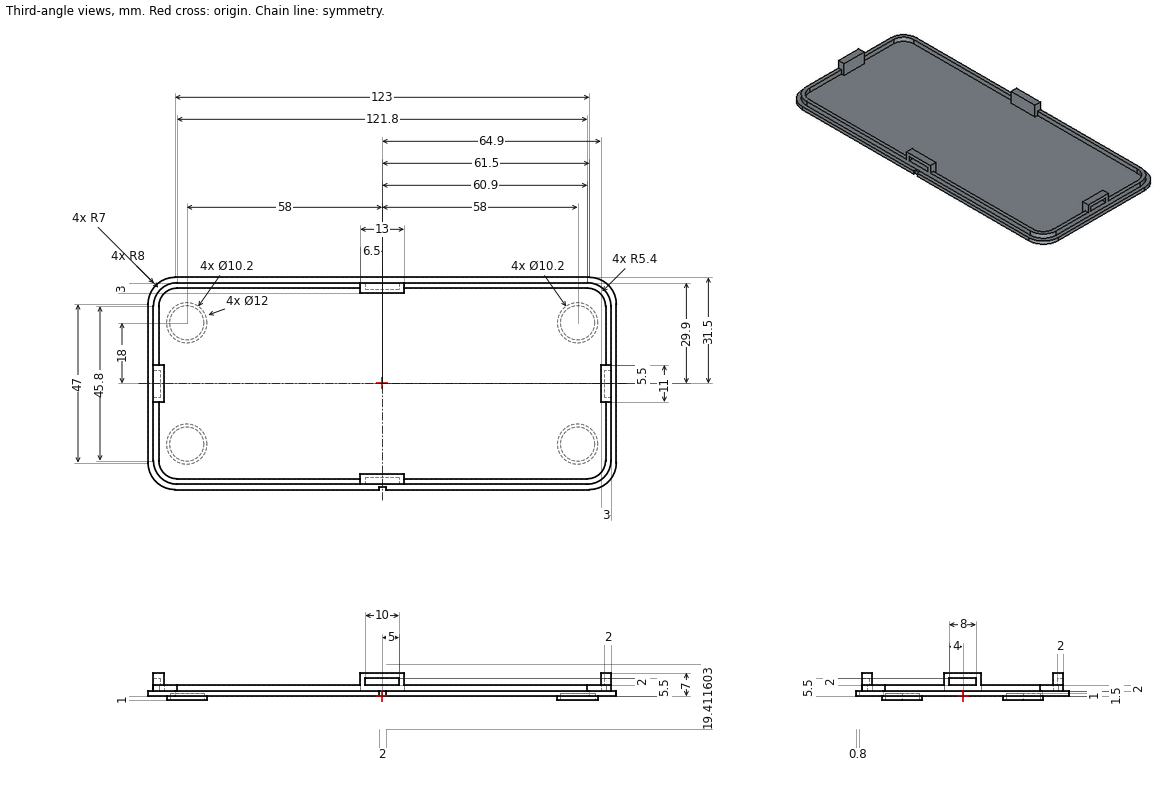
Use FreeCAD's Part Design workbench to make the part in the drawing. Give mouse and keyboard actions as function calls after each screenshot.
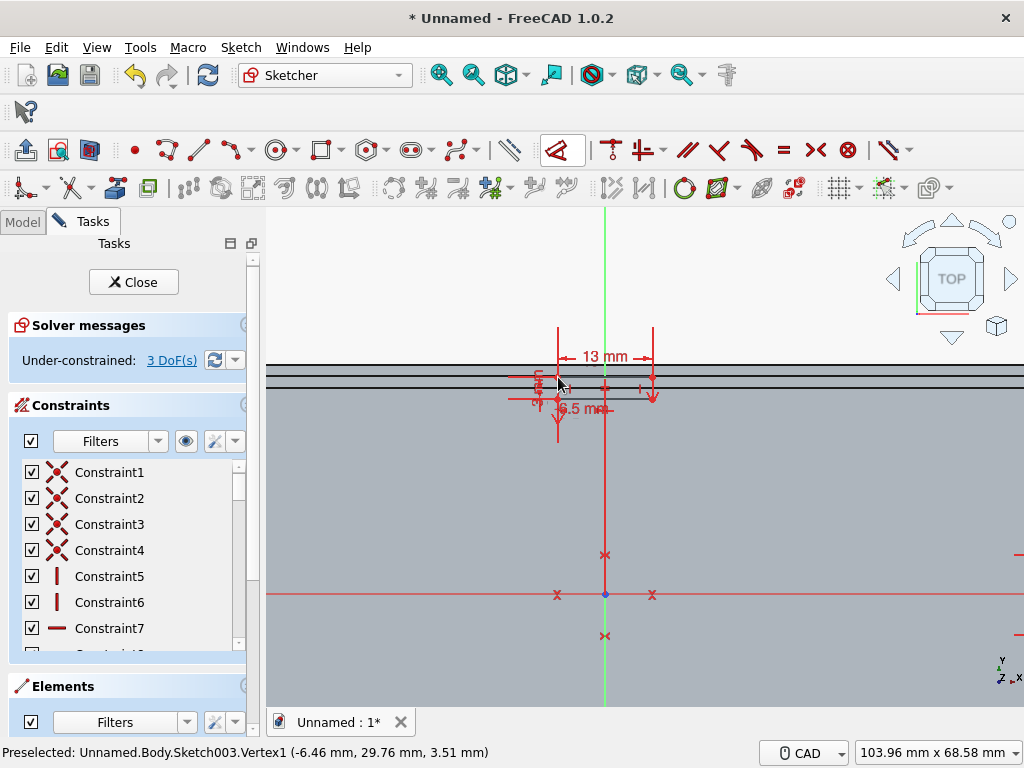
scroll(560, 377, down, 5)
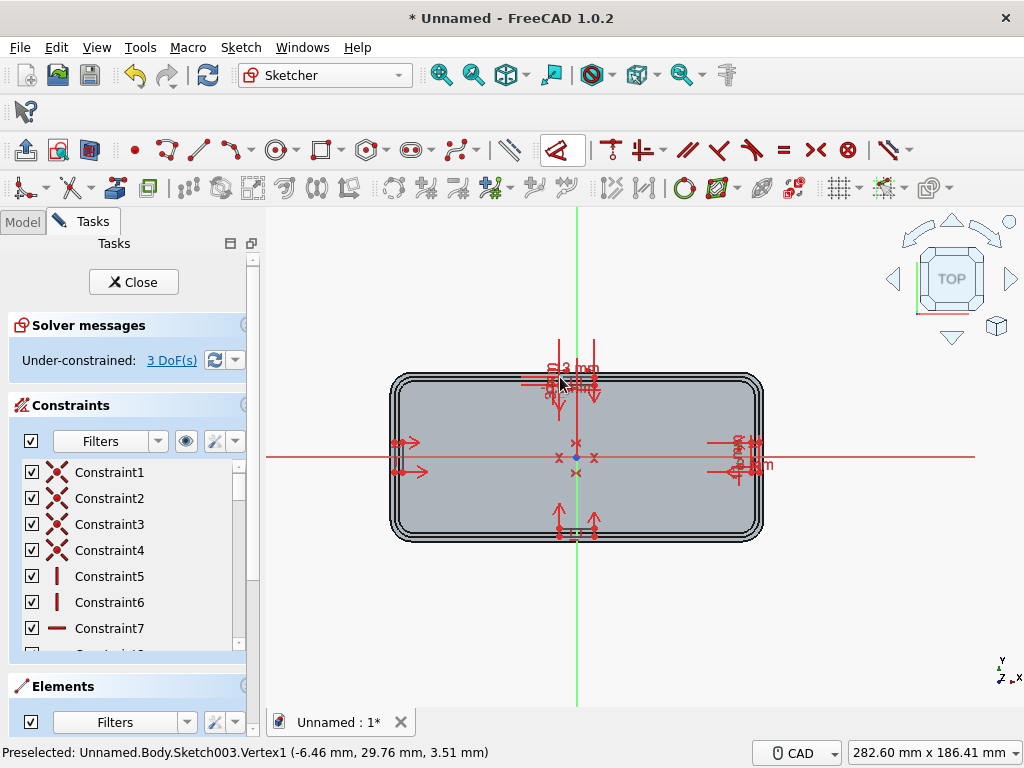
scroll(751, 443, up, 5)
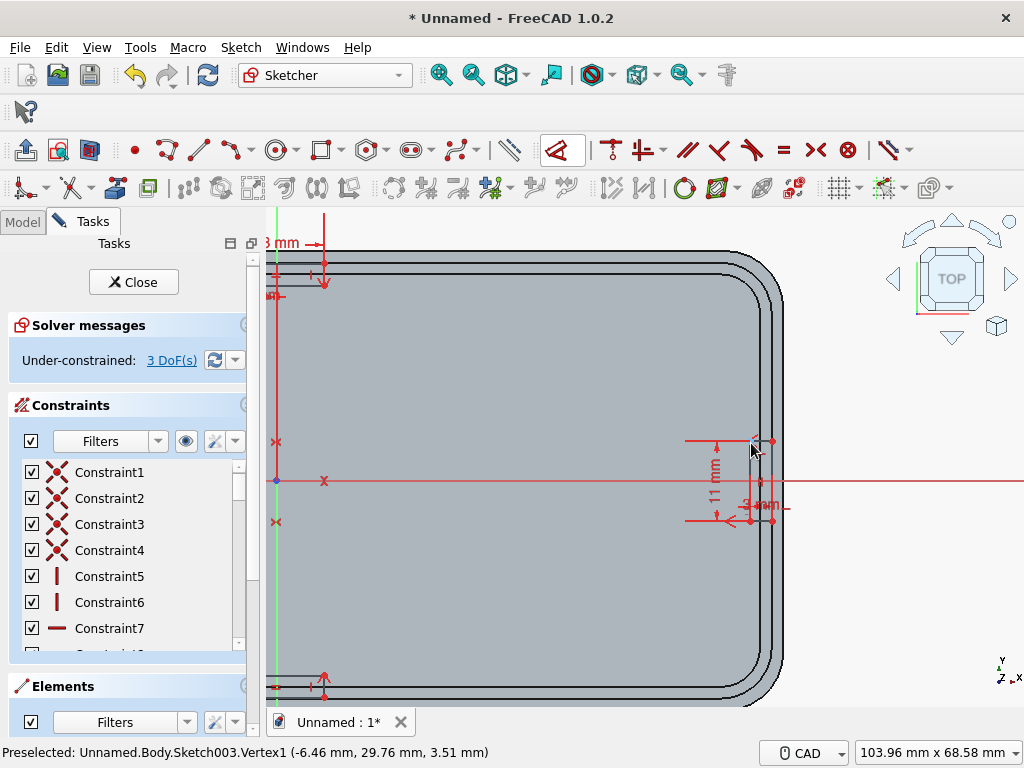
click(750, 441)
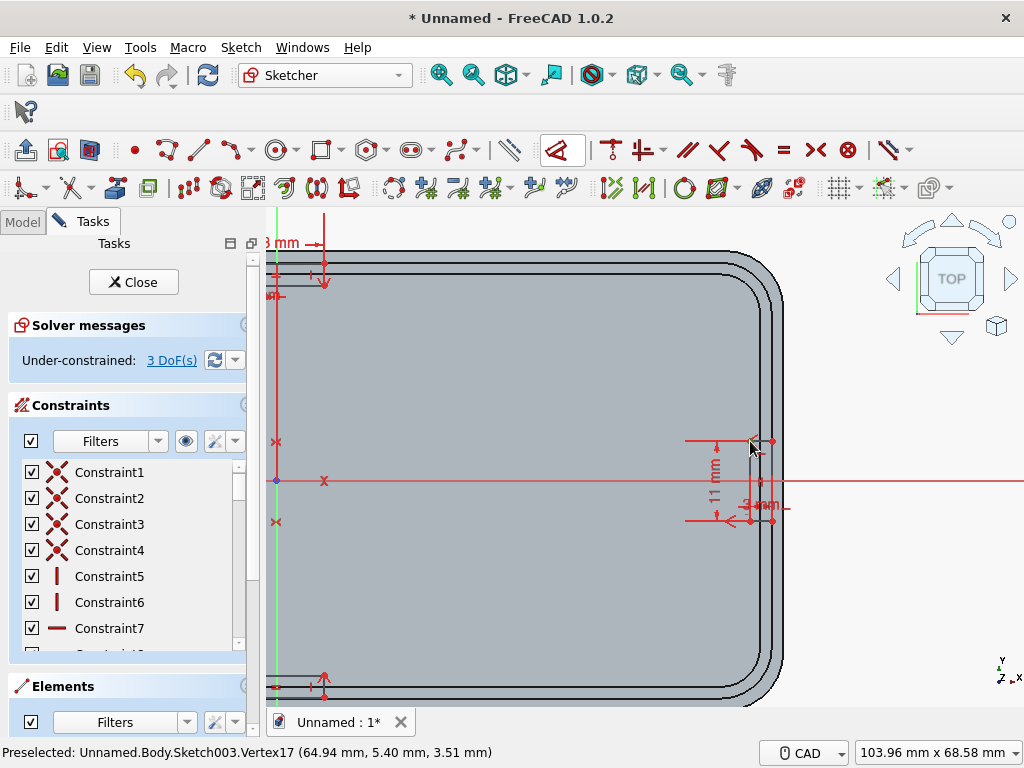
key(i)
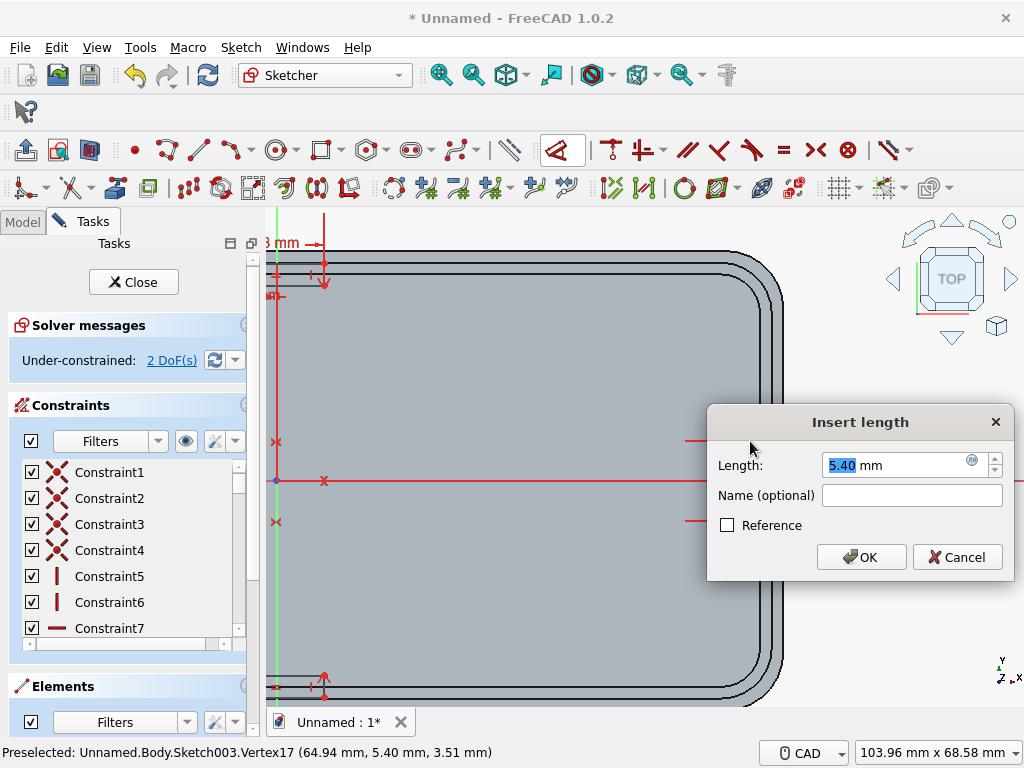
text(5.5)
key(Return)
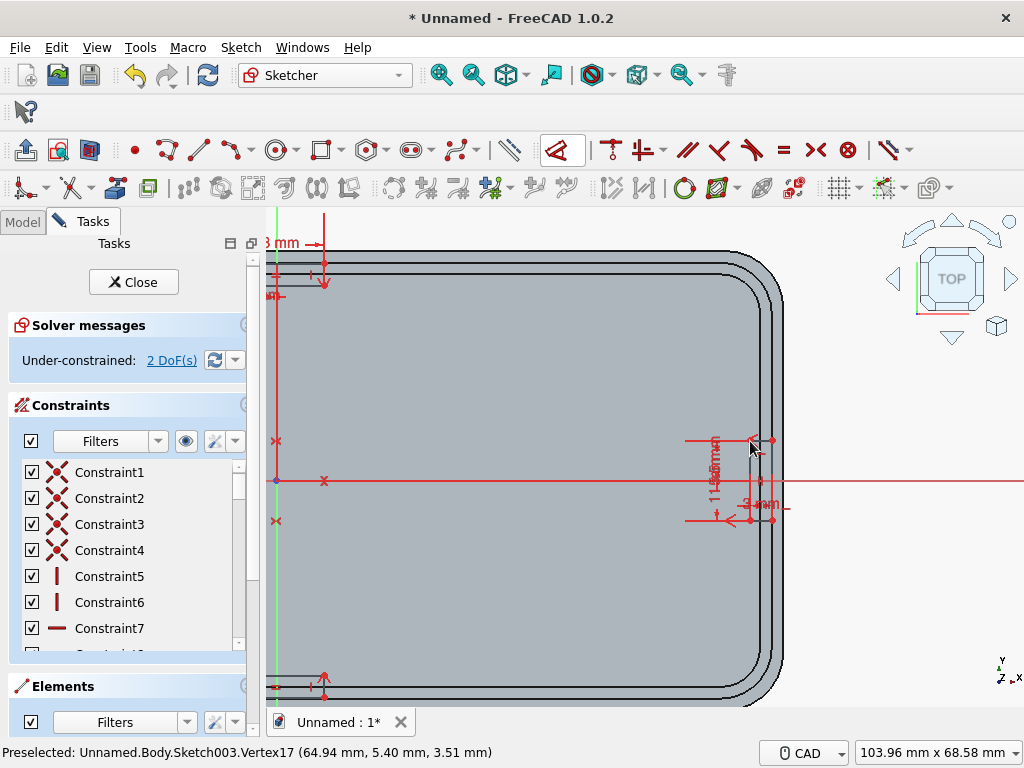
scroll(751, 443, down, 5)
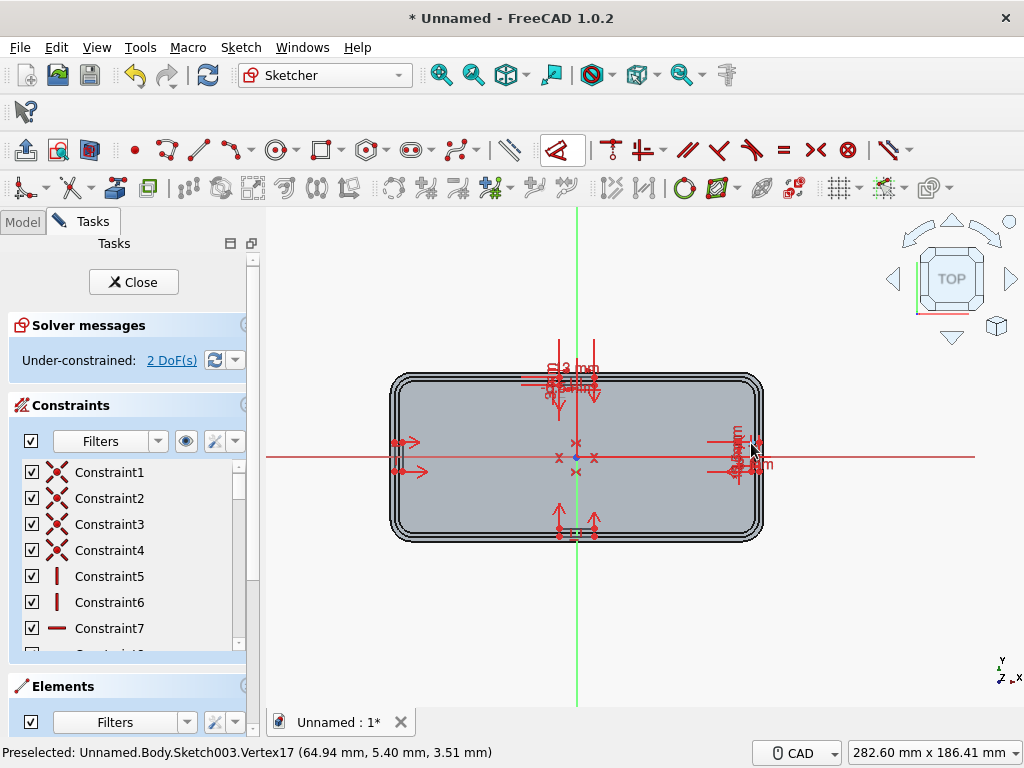
scroll(559, 377, up, 3)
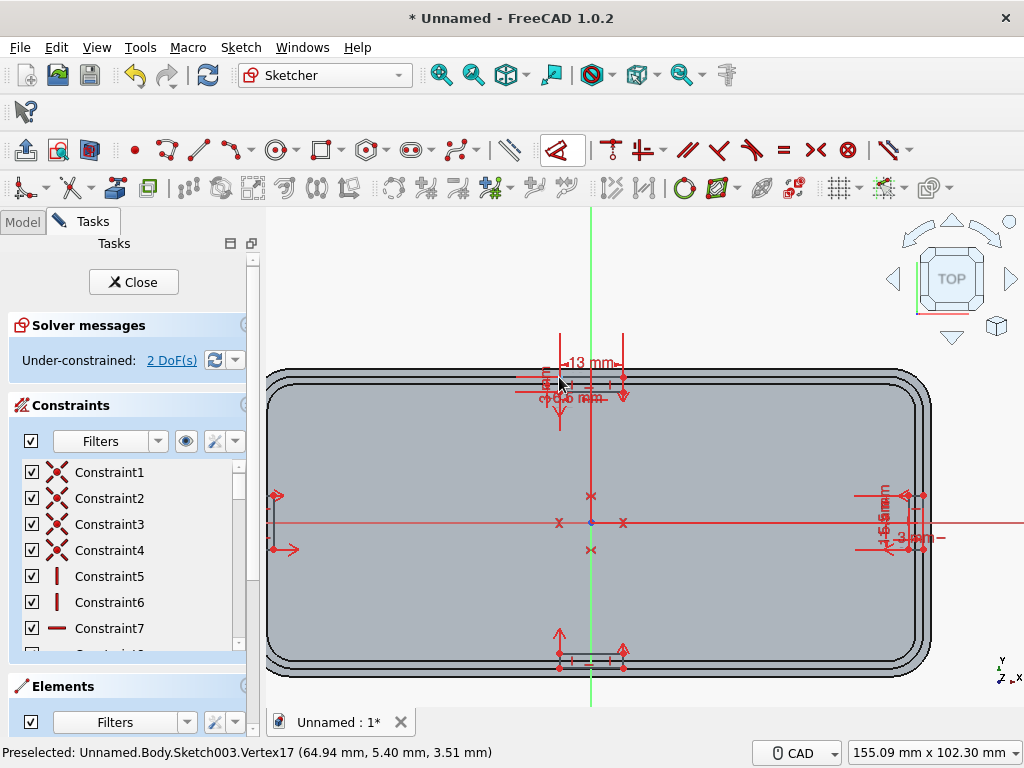
click(560, 377)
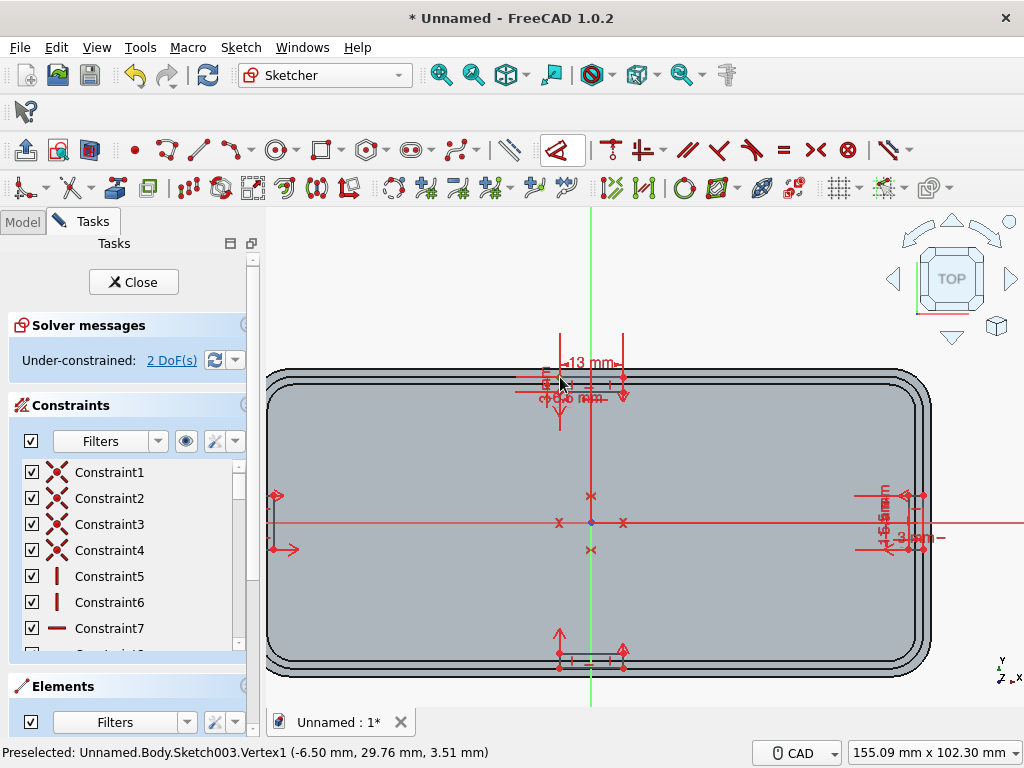
key(i)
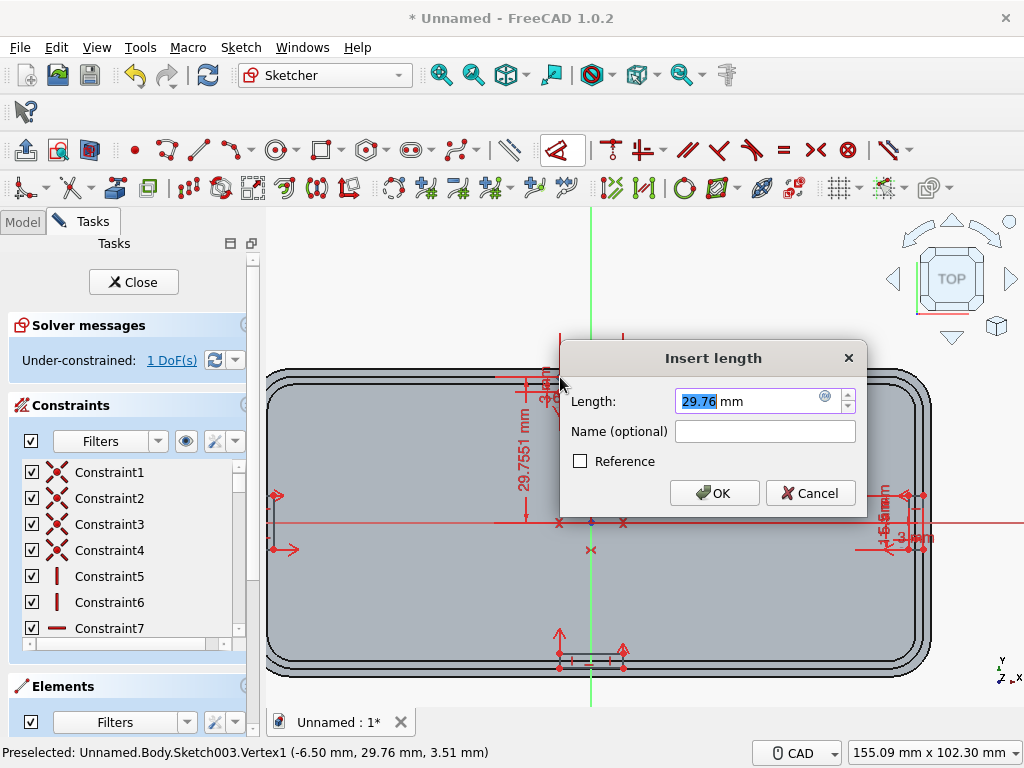
text(29.9)
key(Return)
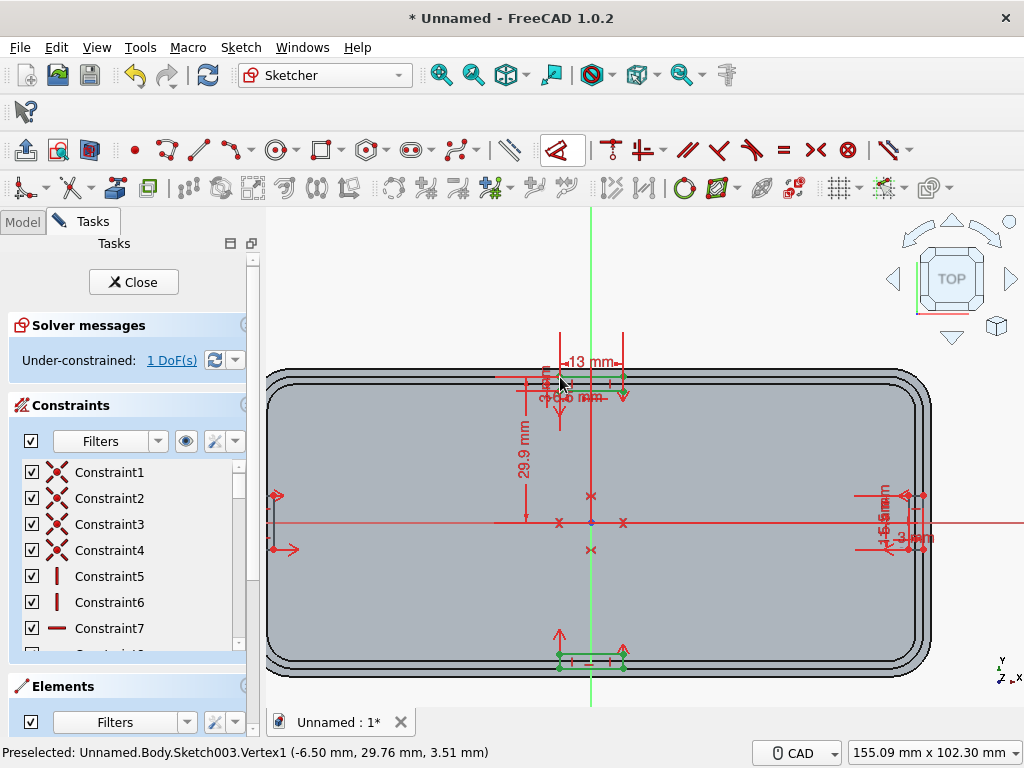
scroll(558, 377, down, 3)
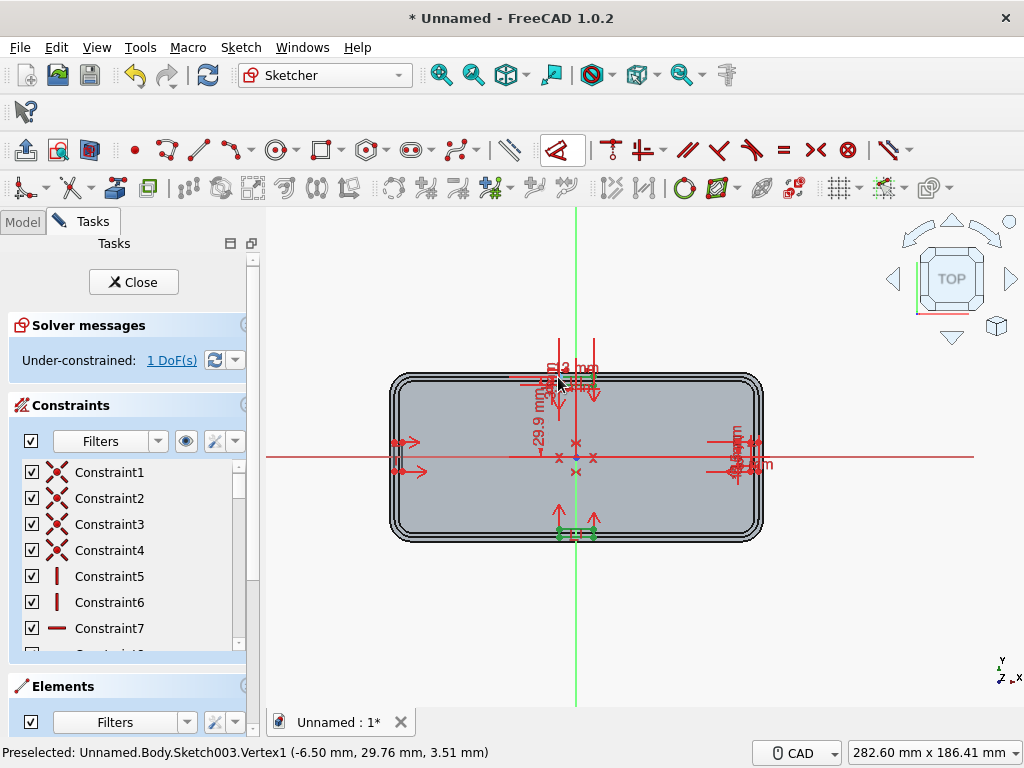
scroll(751, 442, up, 3)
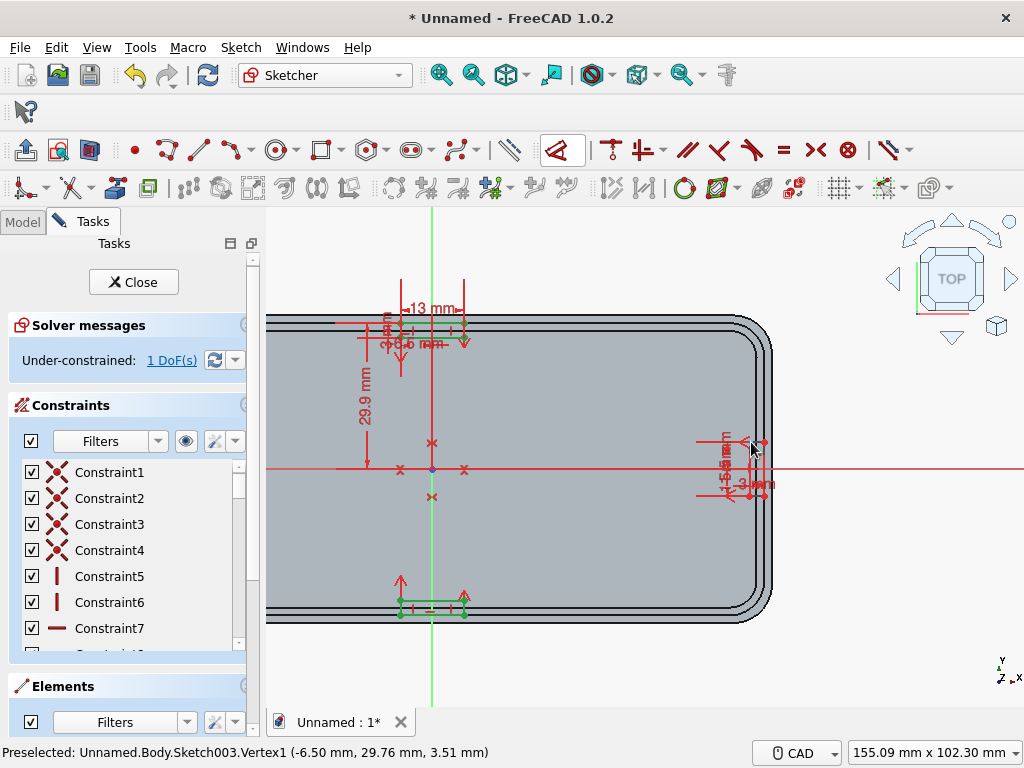
click(750, 442)